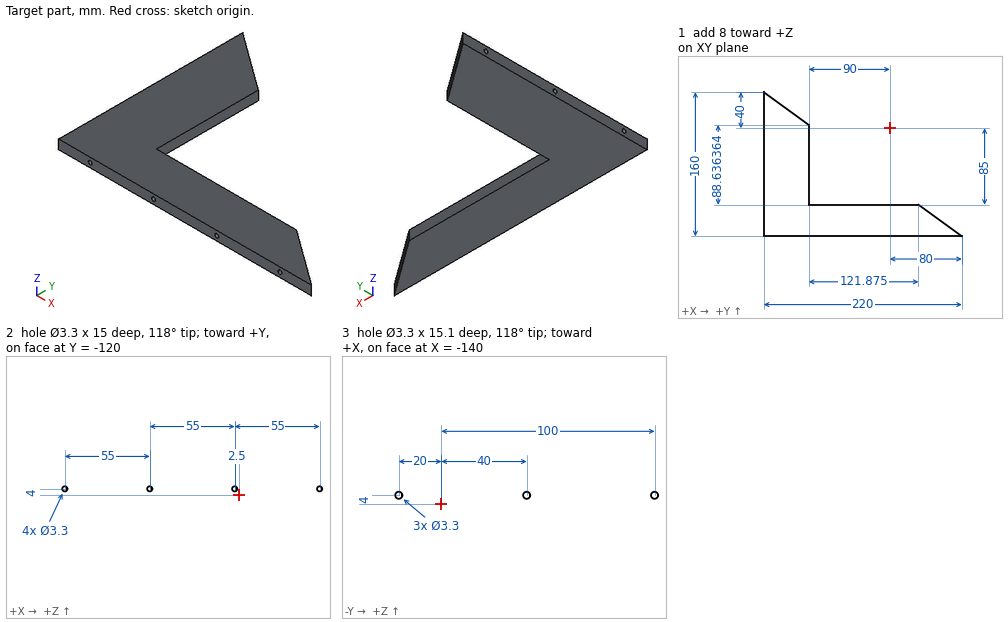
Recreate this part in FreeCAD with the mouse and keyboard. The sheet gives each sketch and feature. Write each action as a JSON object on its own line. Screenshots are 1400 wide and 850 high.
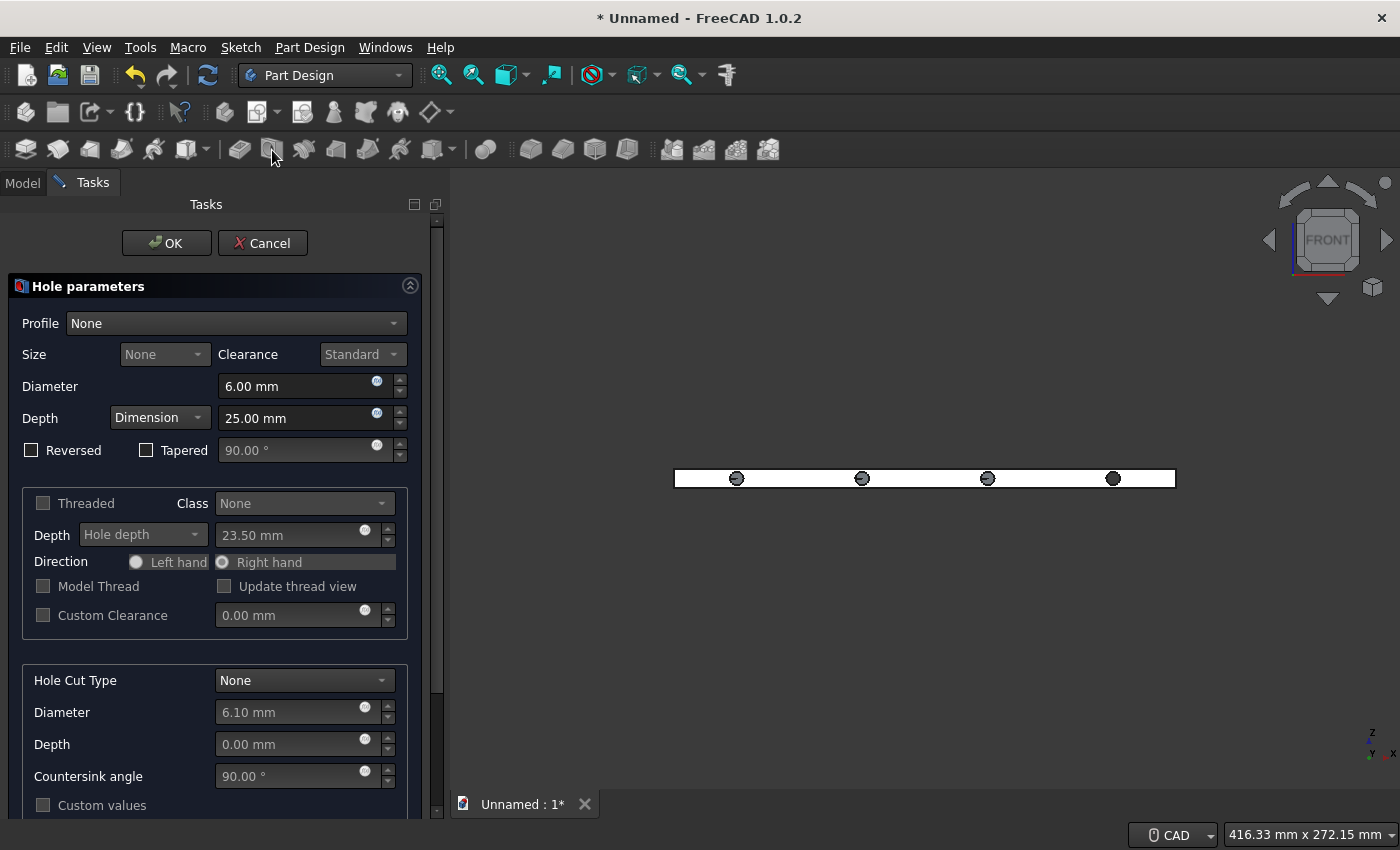
{"action": "triple_click", "coordinate": [305, 386]}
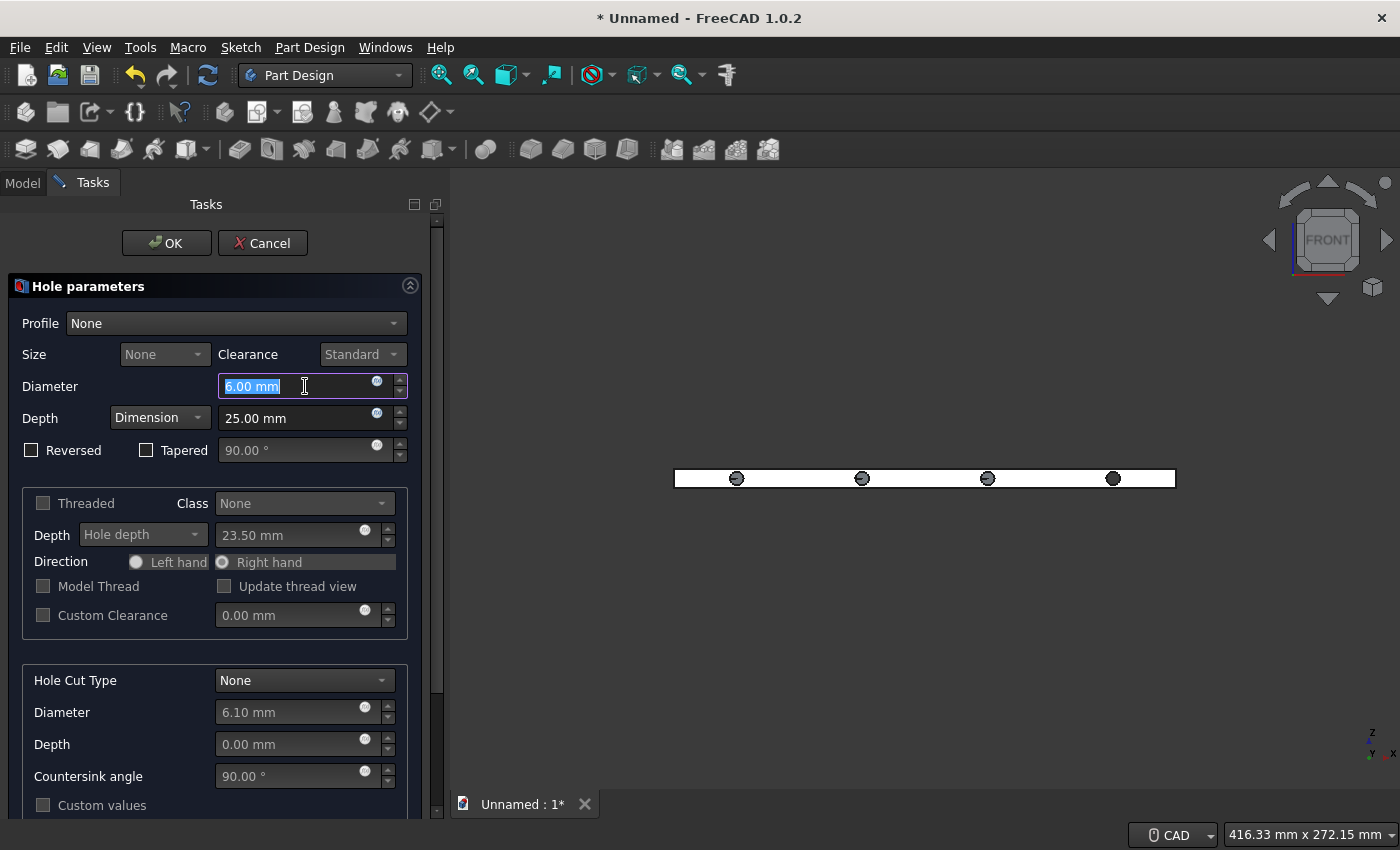
{"action": "type", "text": "3.3"}
{"action": "key", "text": "Tab"}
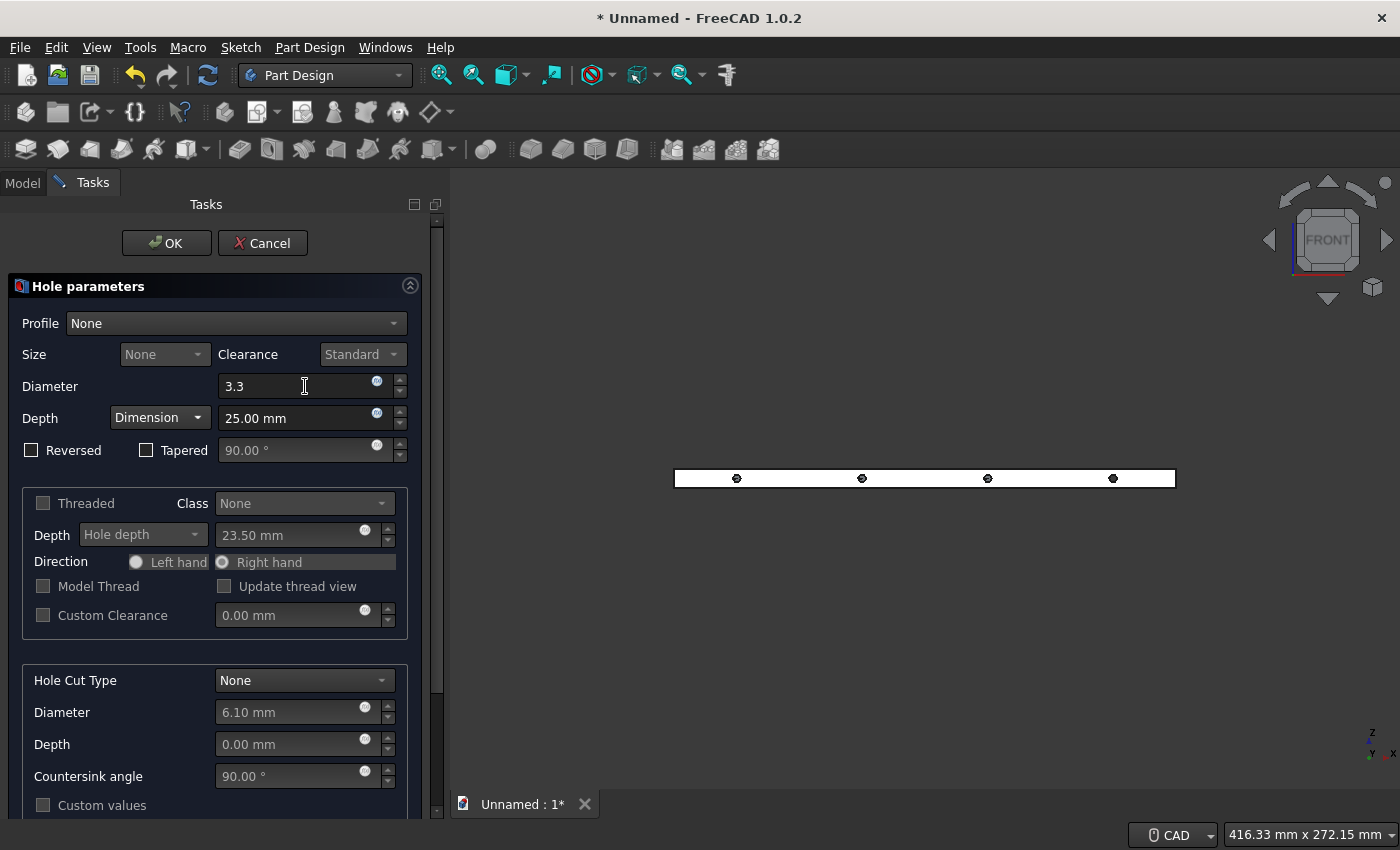
{"action": "triple_click", "coordinate": [305, 418]}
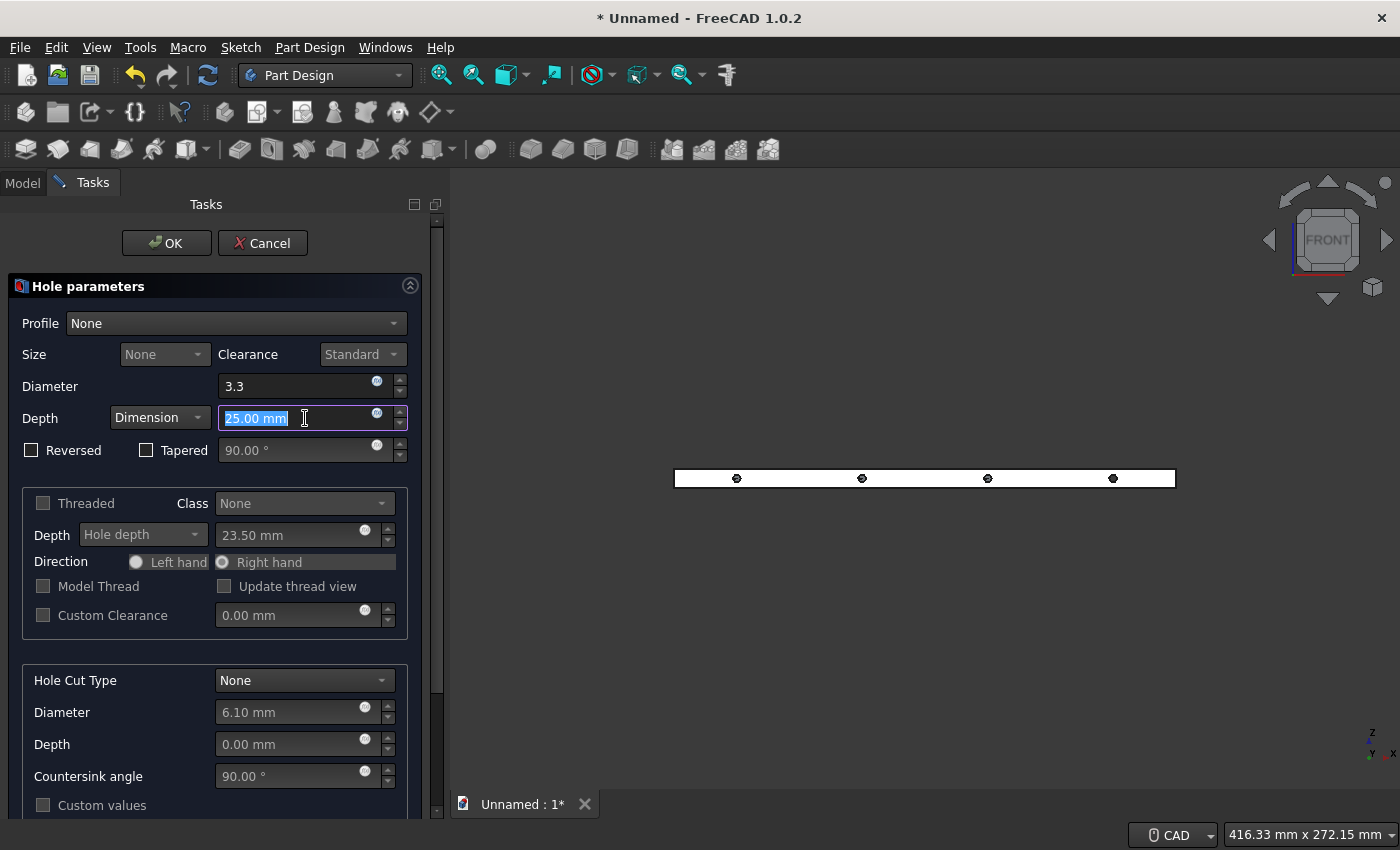
{"action": "type", "text": "15"}
{"action": "key", "text": "Tab"}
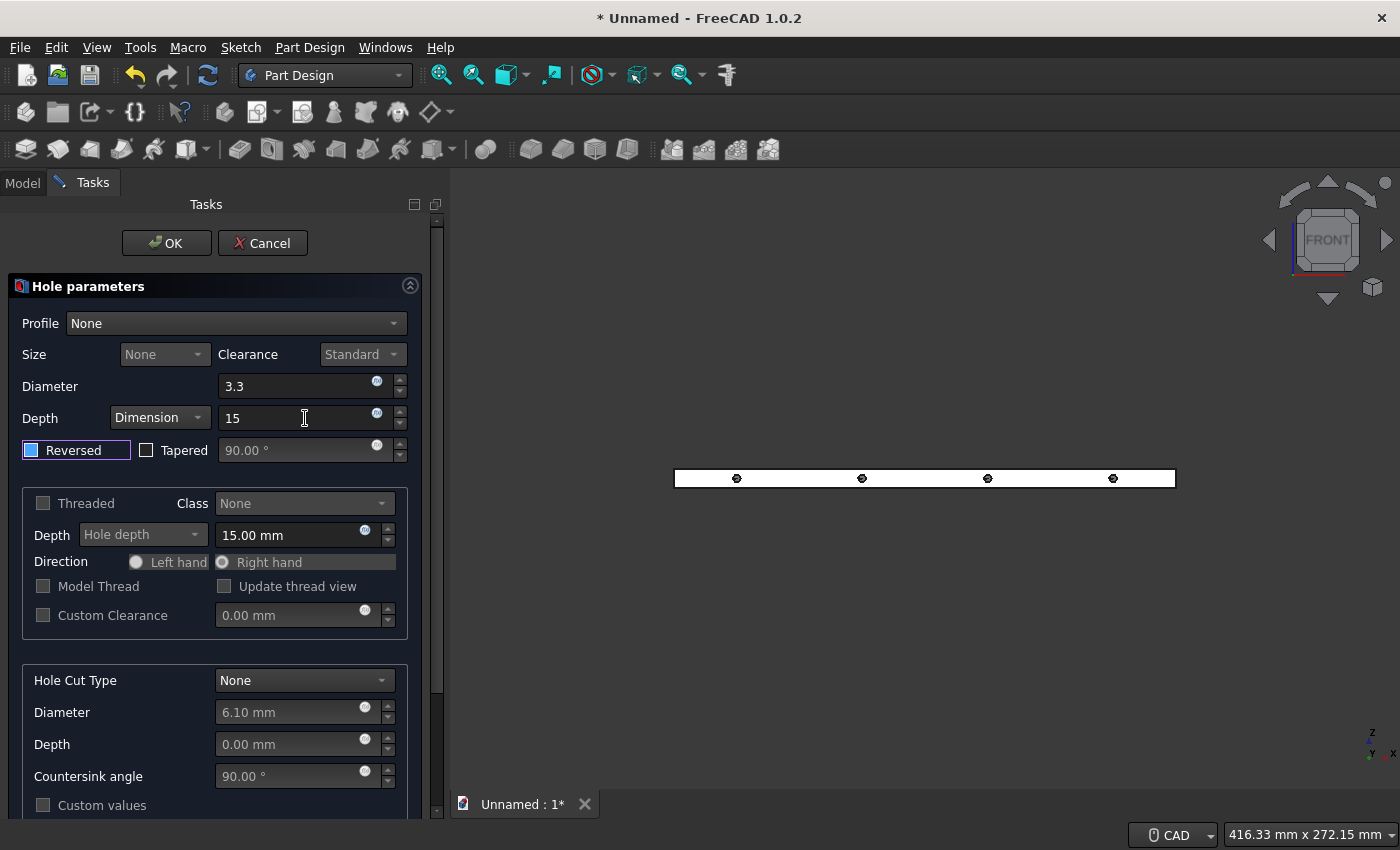
{"action": "left_click", "coordinate": [167, 243]}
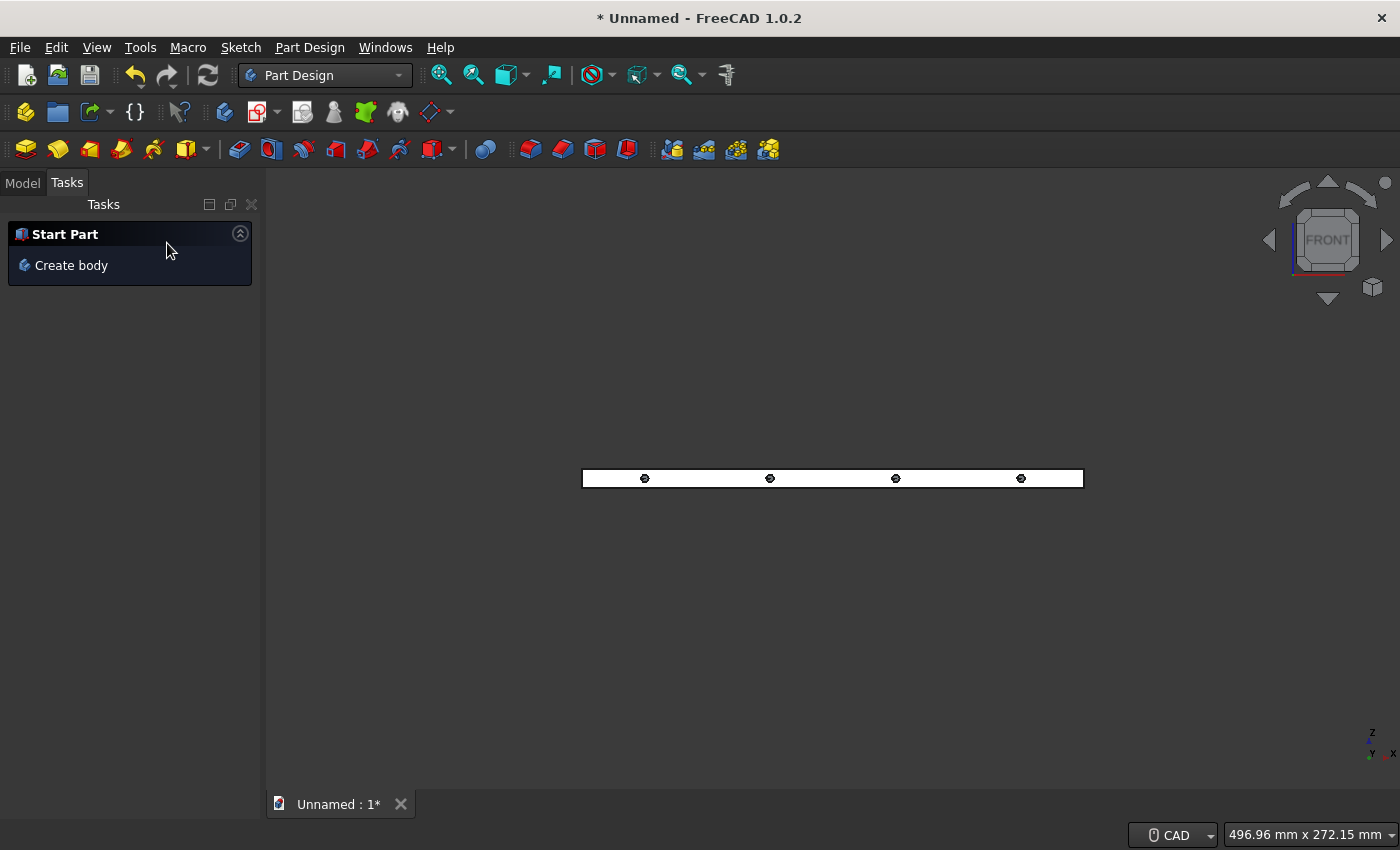
{"action": "key", "text": "v f"}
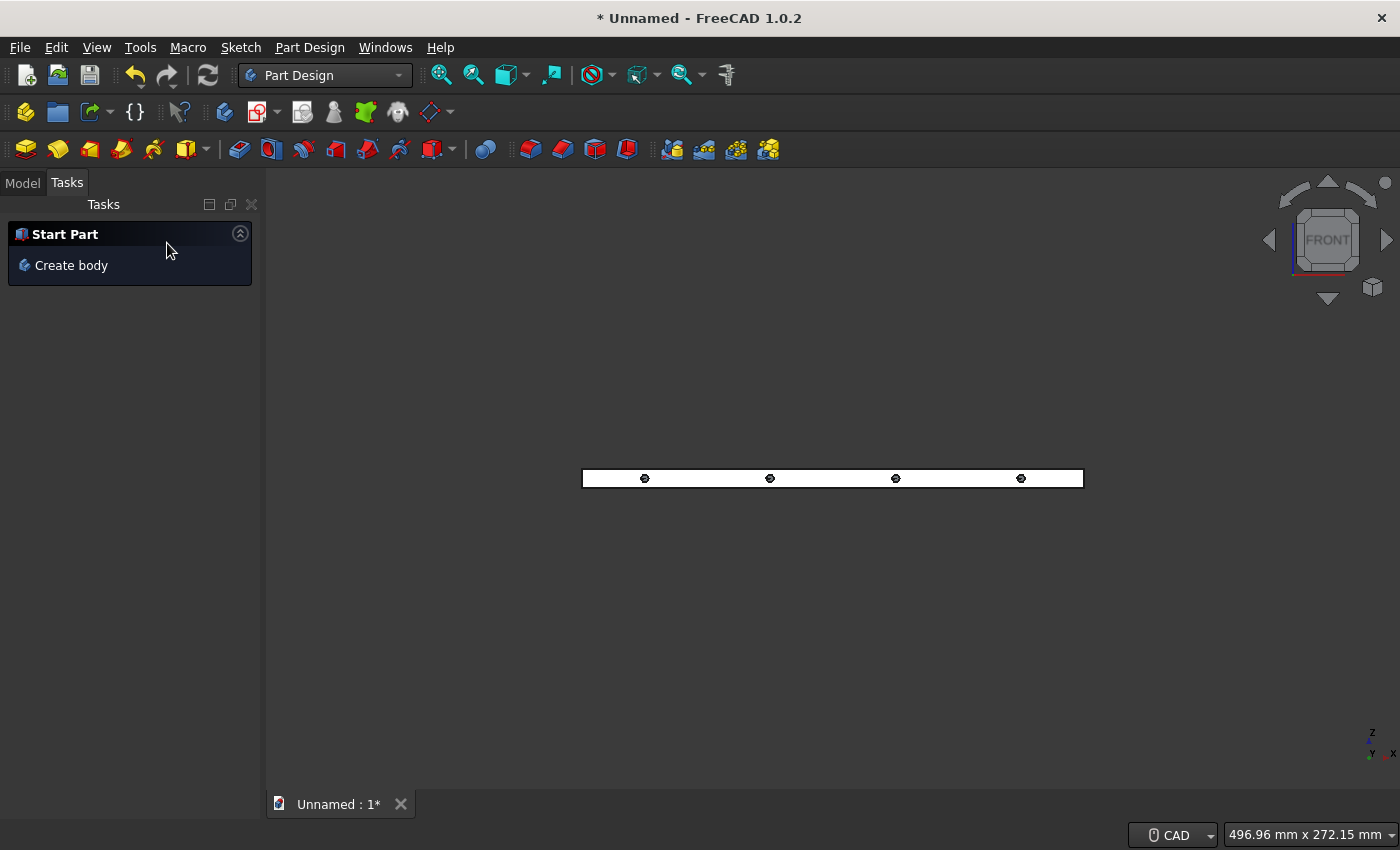
{"action": "key", "text": "6"}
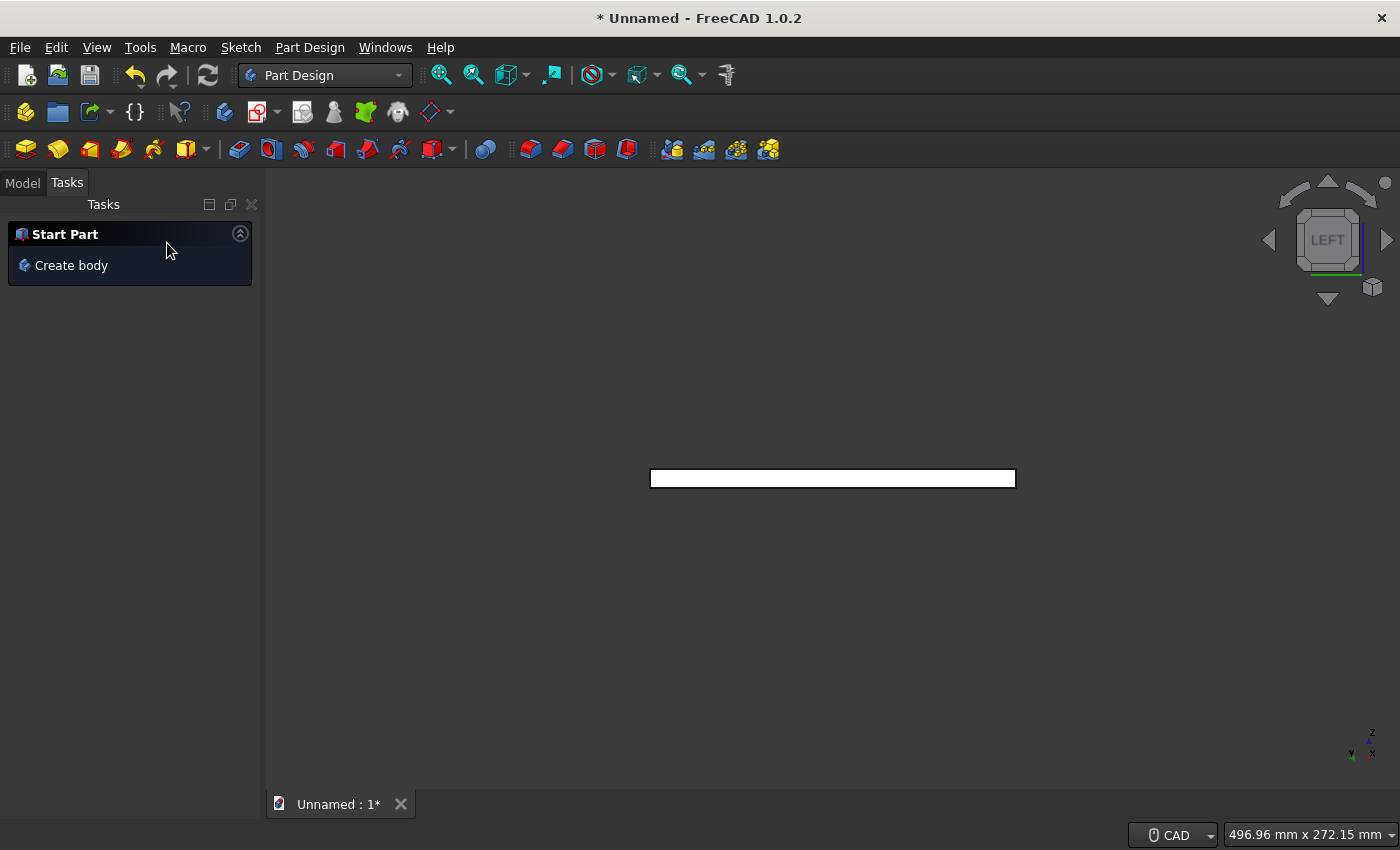
{"action": "key", "text": "v f"}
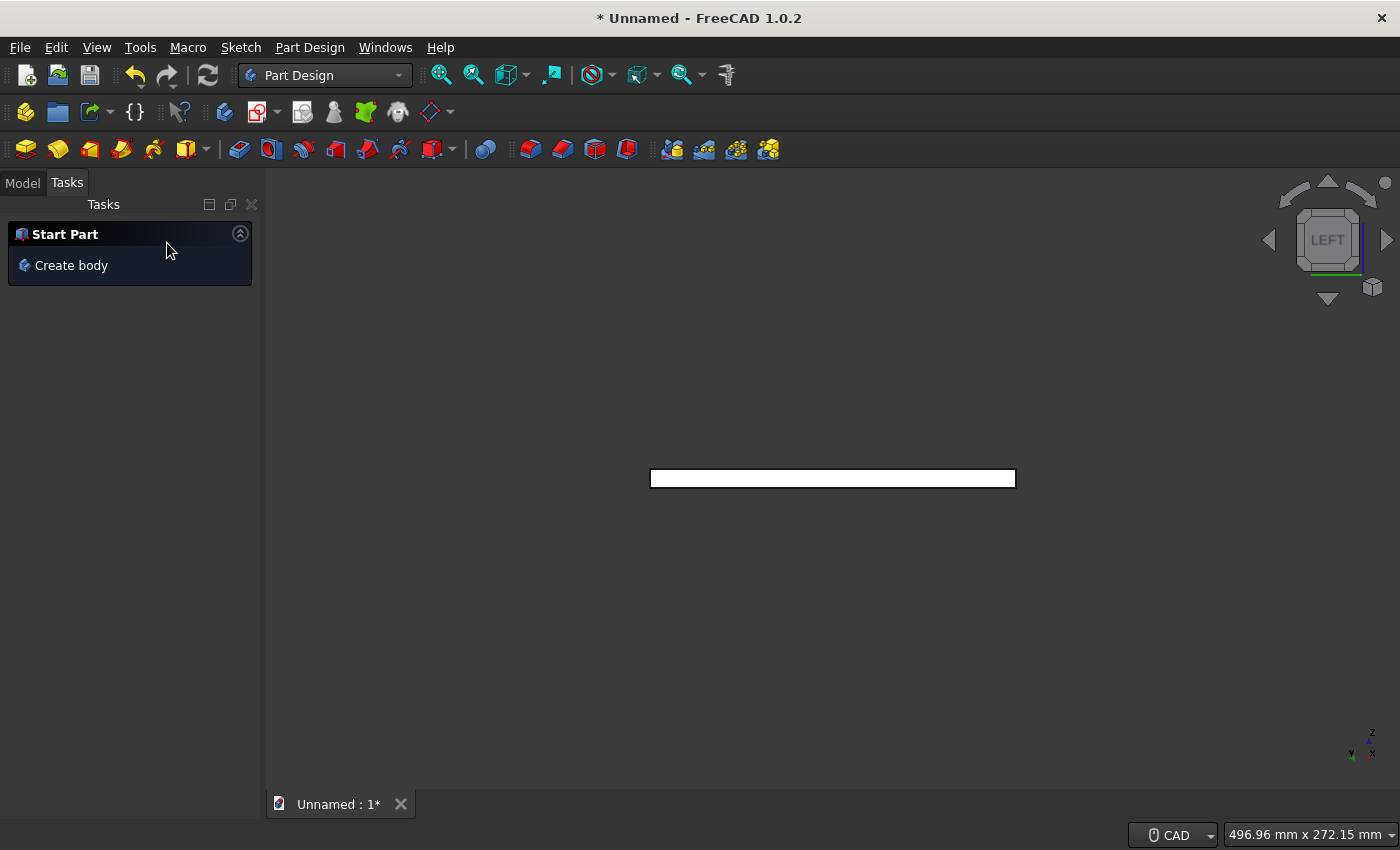
{"action": "left_click", "coordinate": [677, 477]}